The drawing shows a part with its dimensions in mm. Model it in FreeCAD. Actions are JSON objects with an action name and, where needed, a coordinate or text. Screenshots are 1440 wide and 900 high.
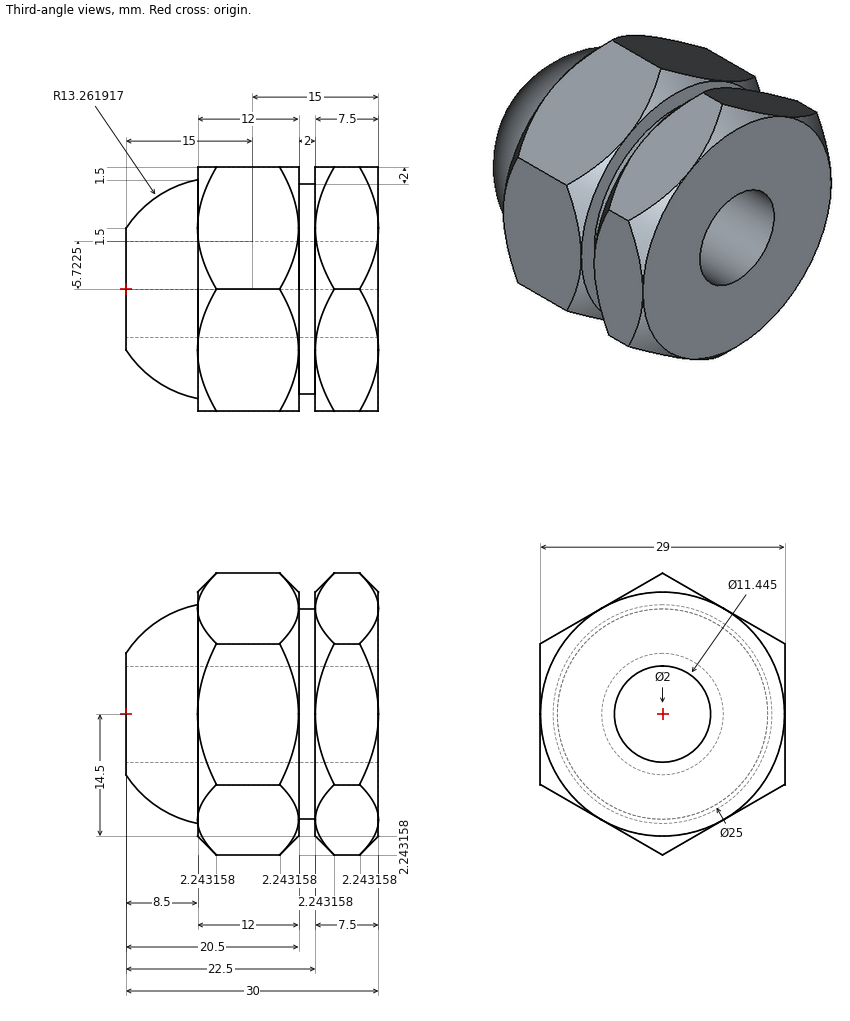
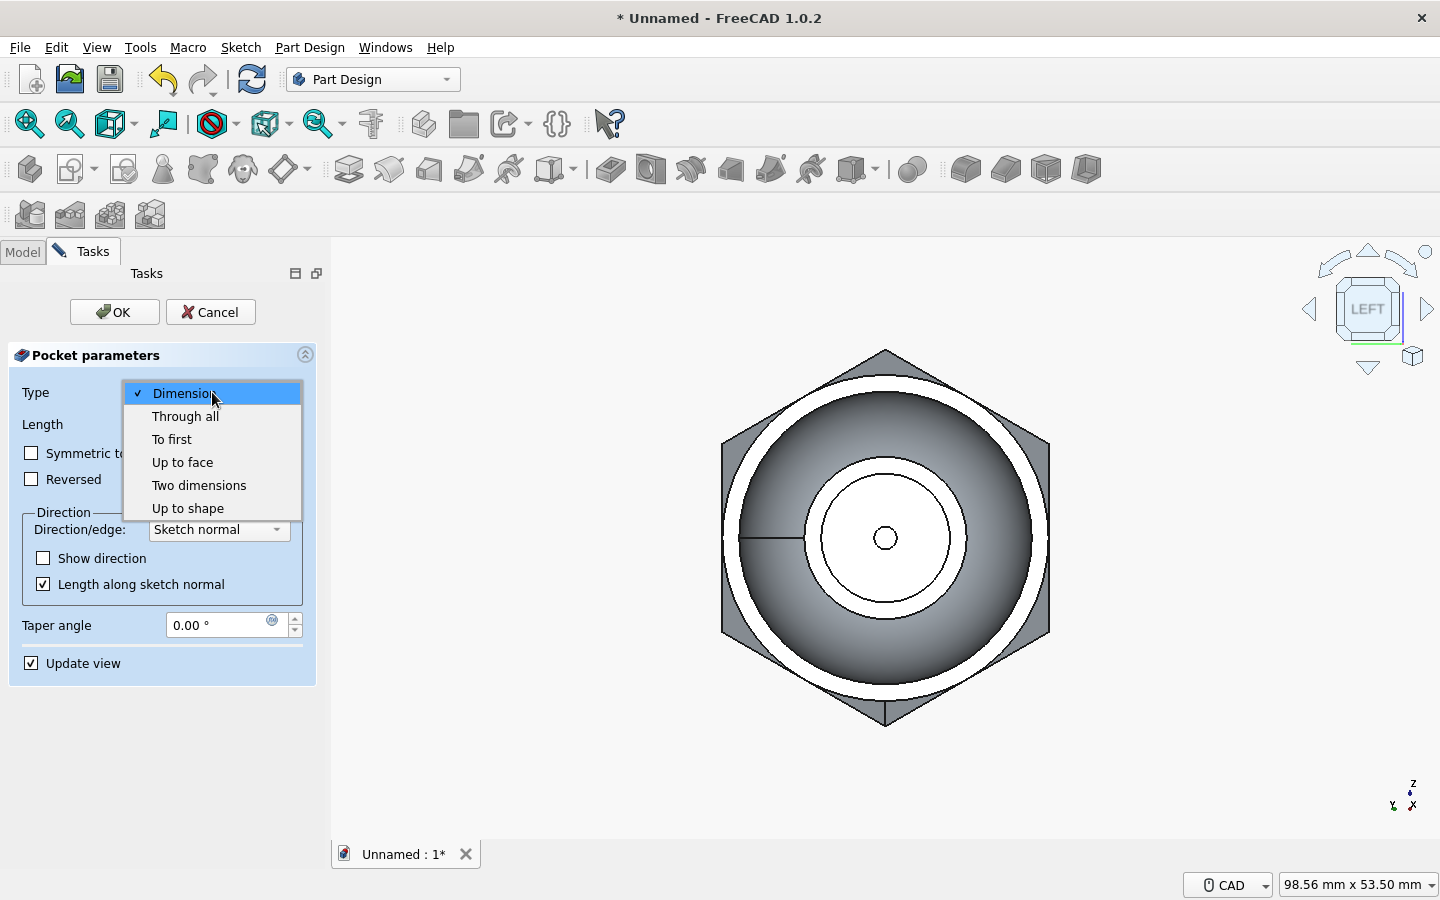
{"action": "left_click", "coordinate": [212, 416]}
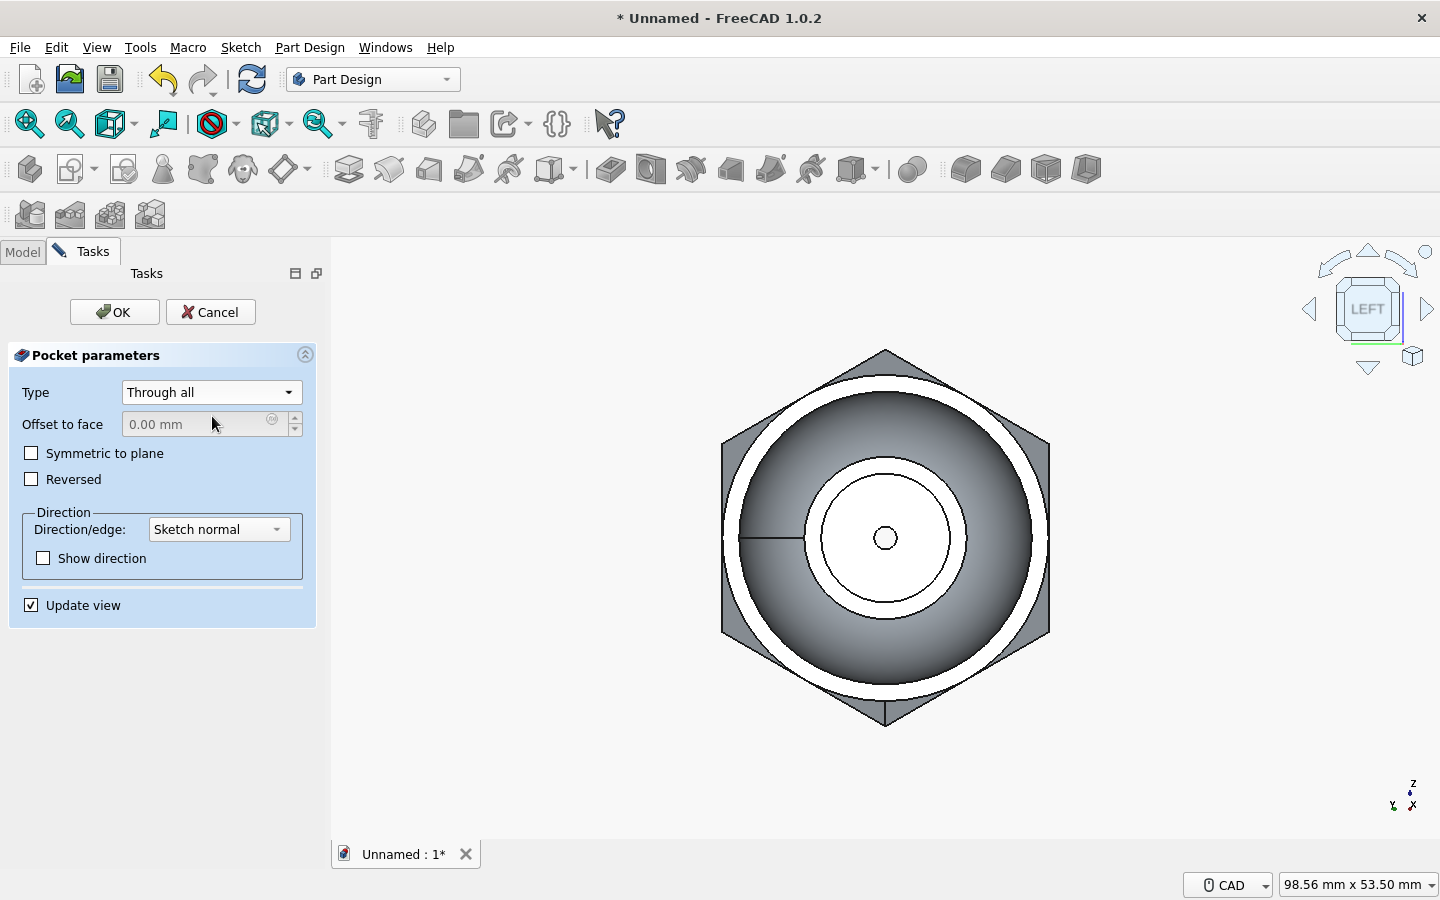
{"action": "left_click", "coordinate": [115, 312]}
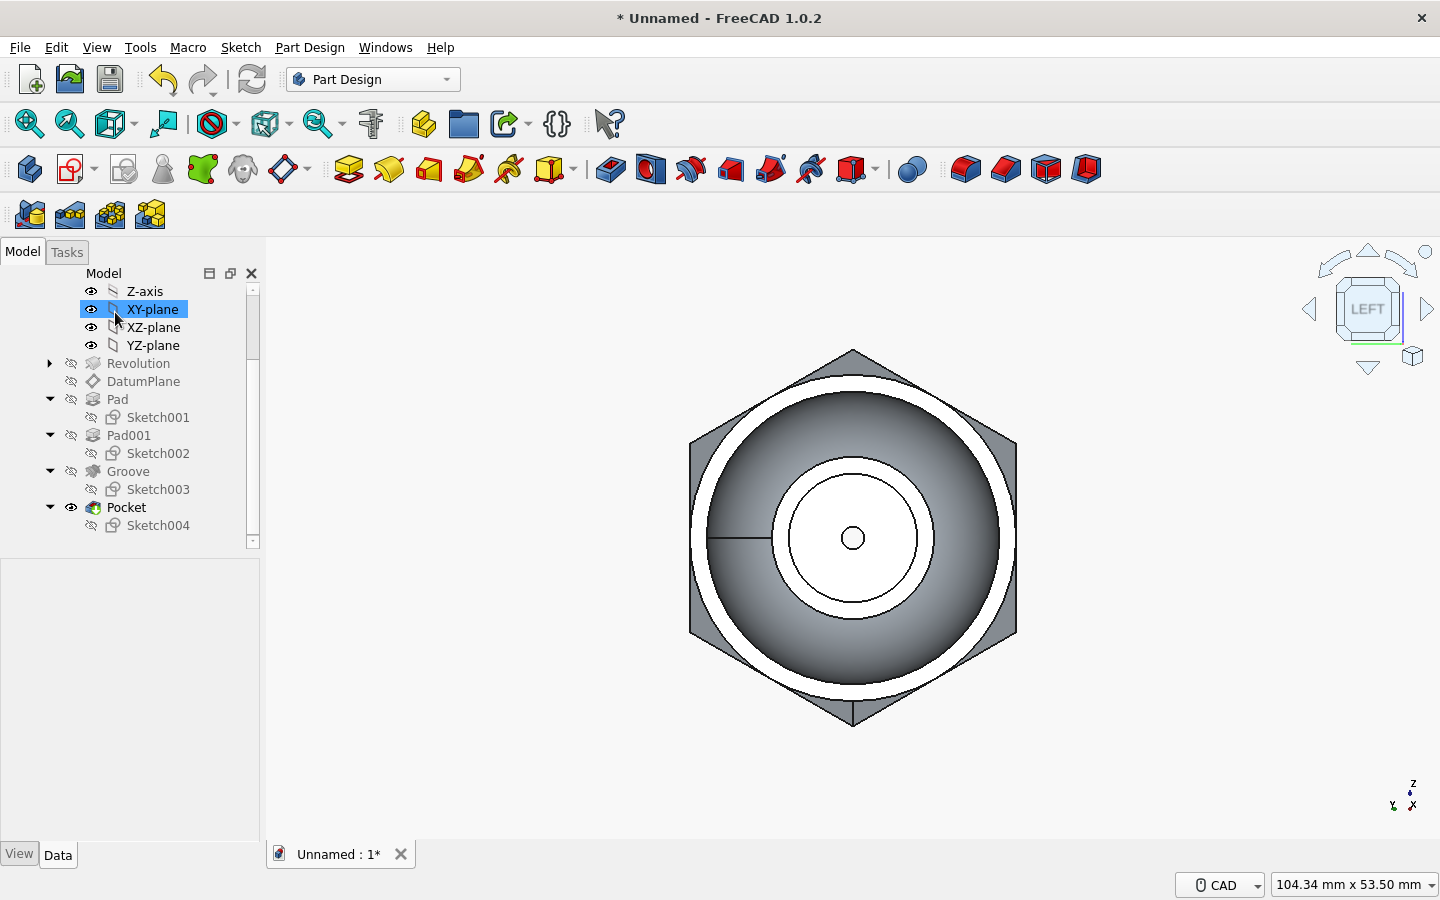
{"action": "left_click", "coordinate": [816, 537]}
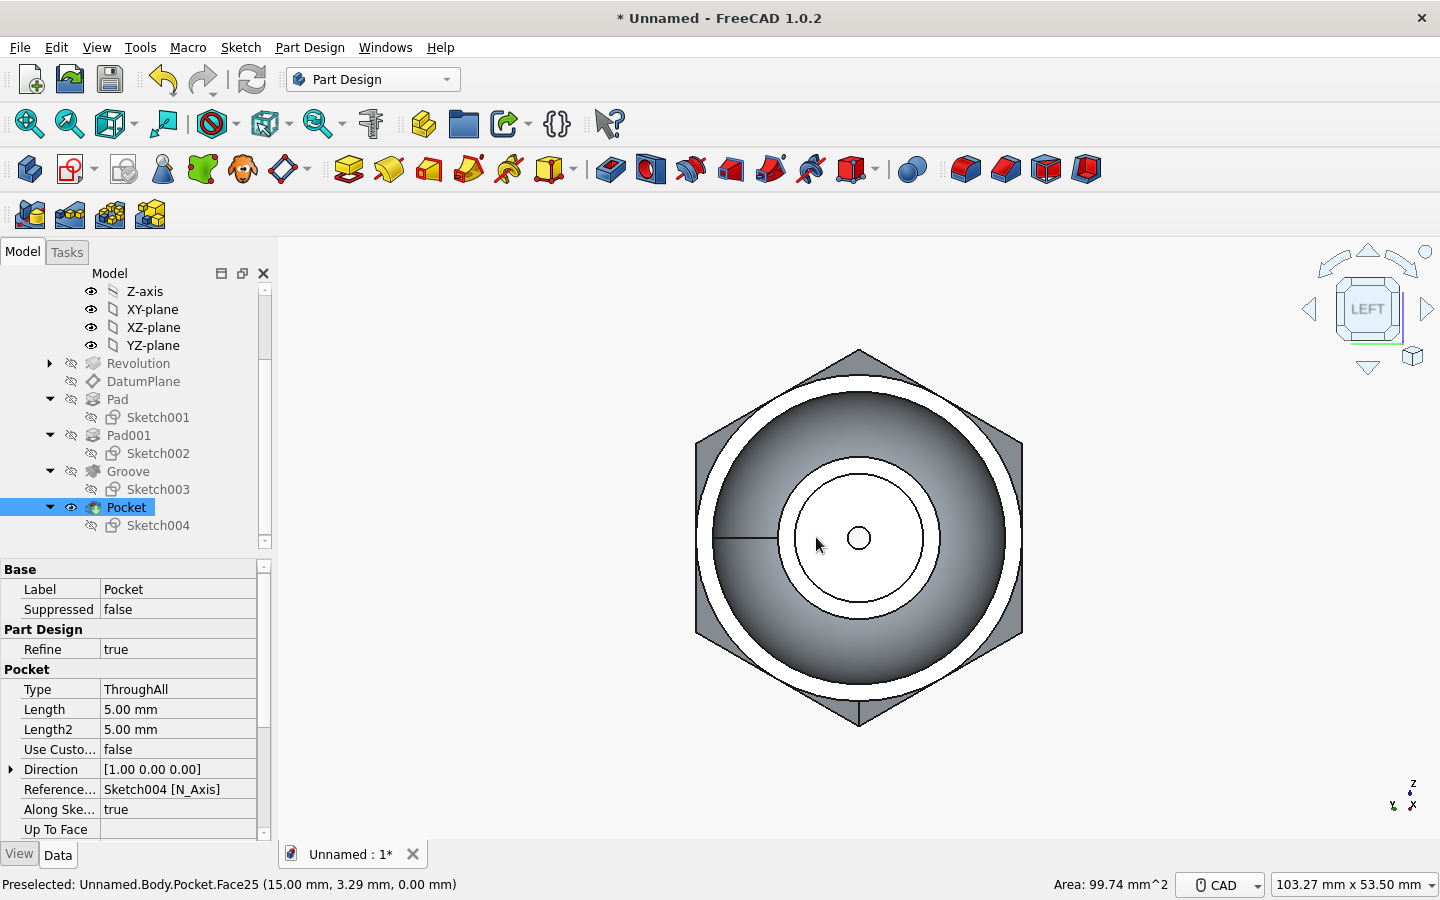
{"action": "left_click", "coordinate": [70, 170]}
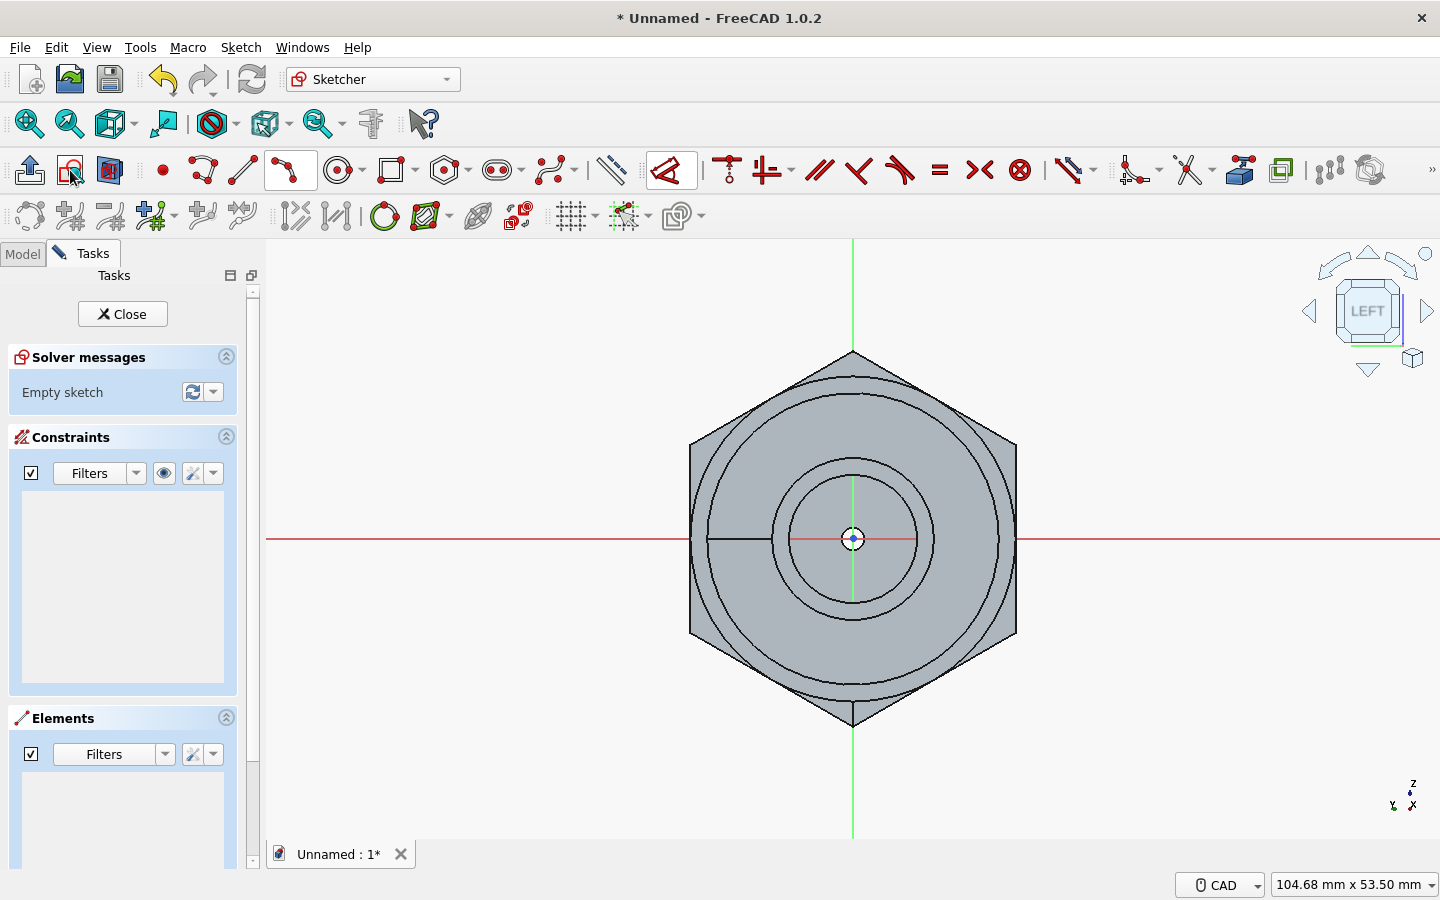
{"action": "left_click", "coordinate": [110, 170]}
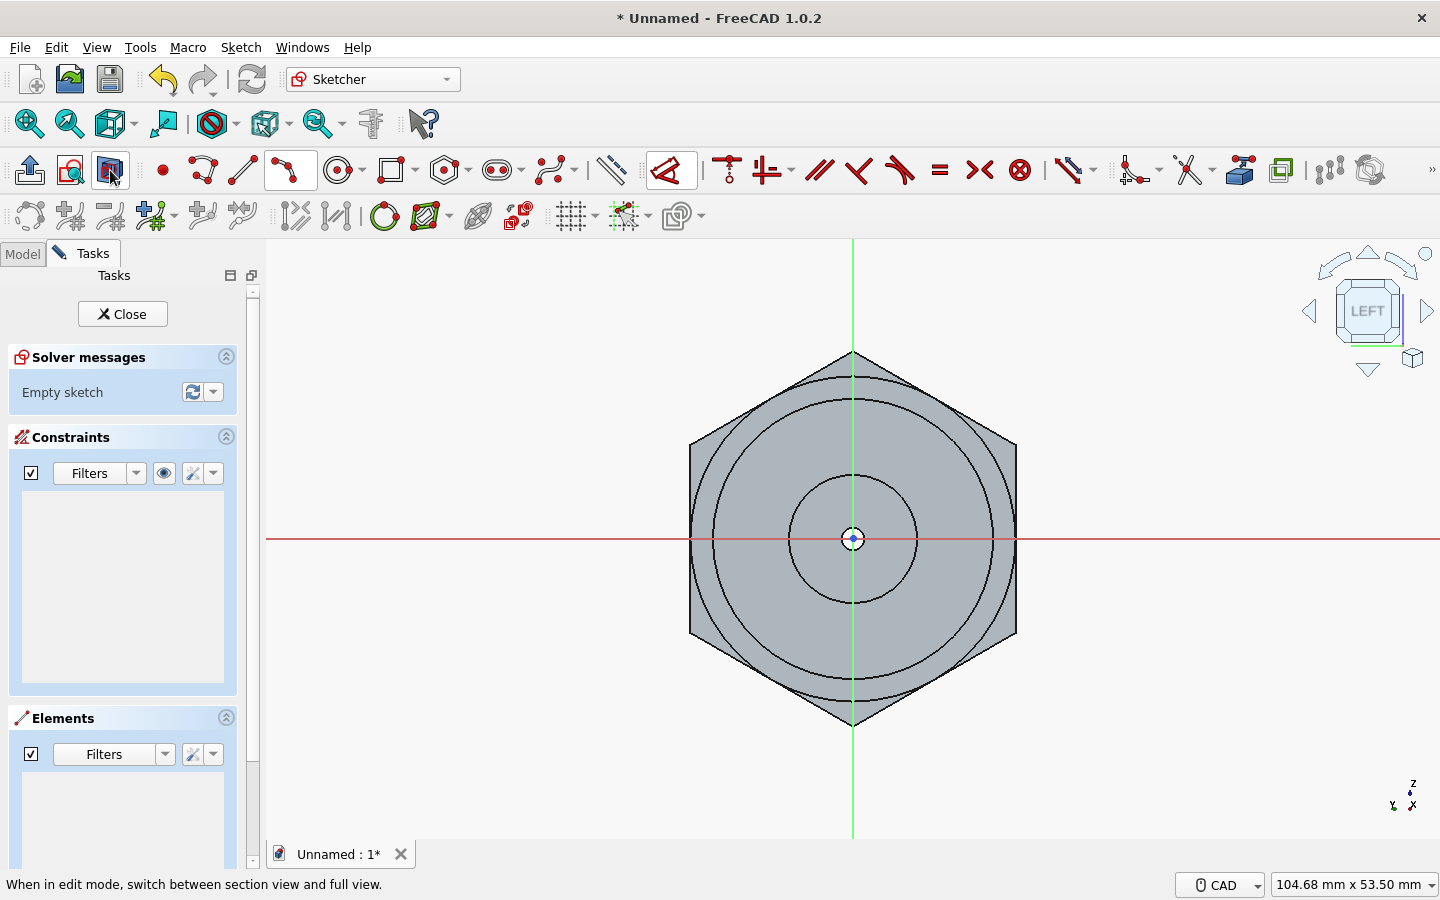
{"action": "scroll", "coordinate": [893, 539], "scroll_direction": "up", "scroll_amount": 5}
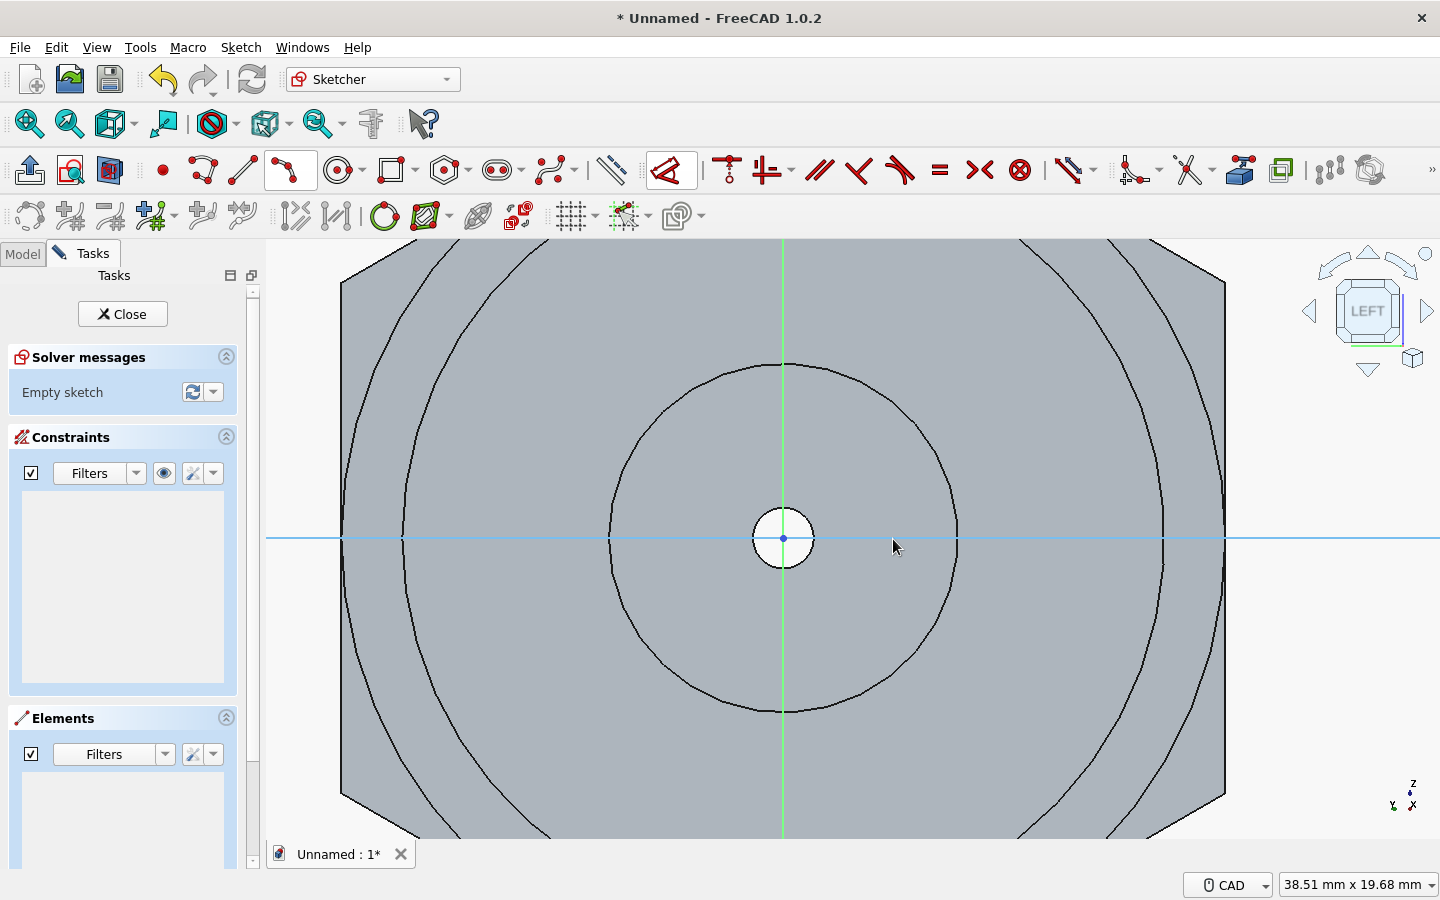
{"action": "left_click", "coordinate": [338, 170]}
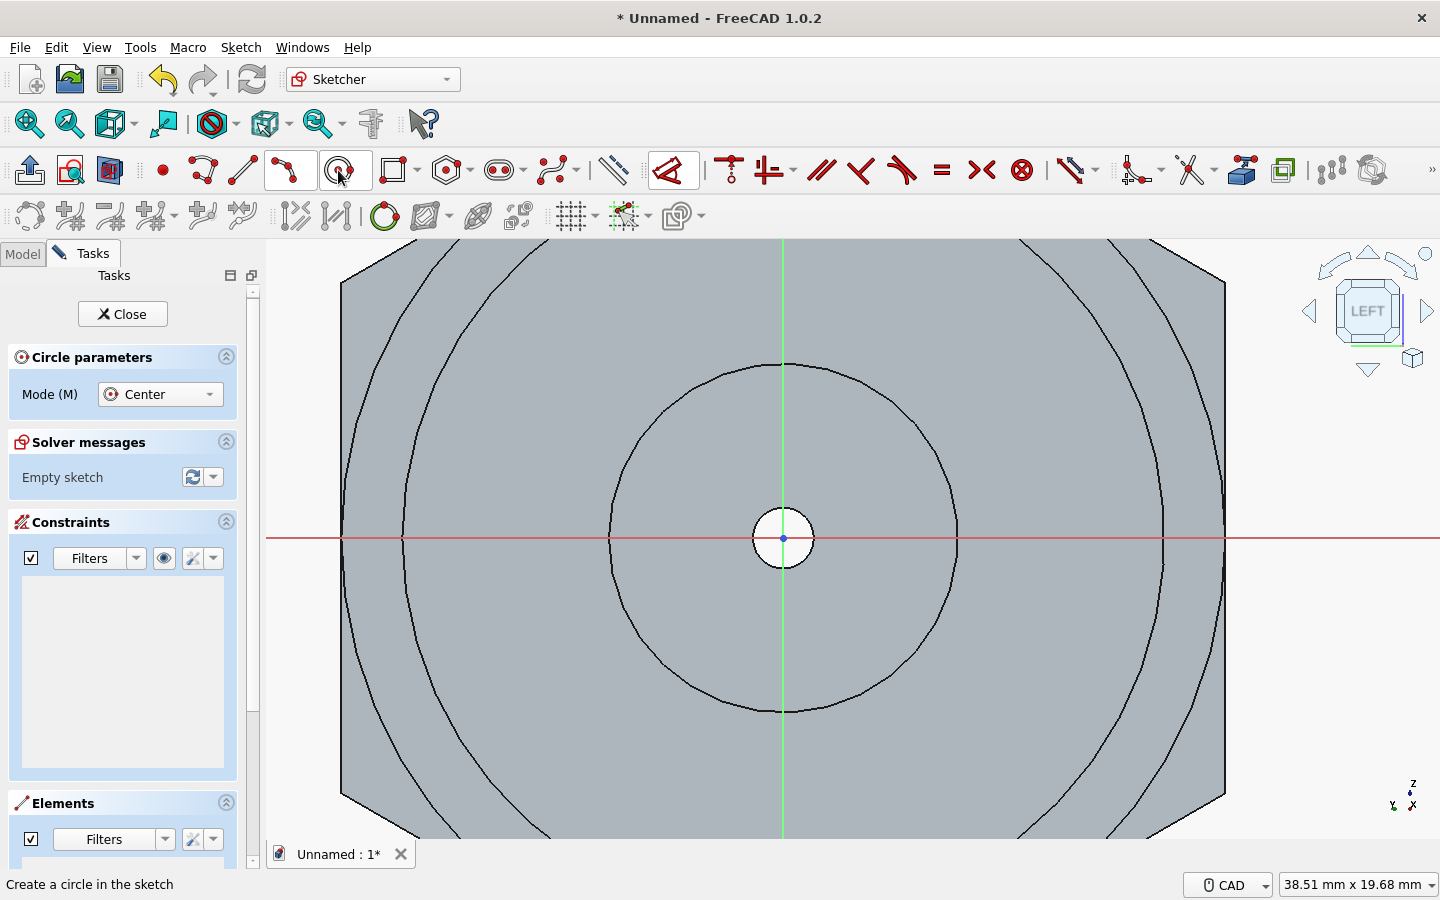
{"action": "left_click", "coordinate": [783, 538]}
{"action": "left_click", "coordinate": [907, 415]}
{"action": "key", "text": "Escape"}